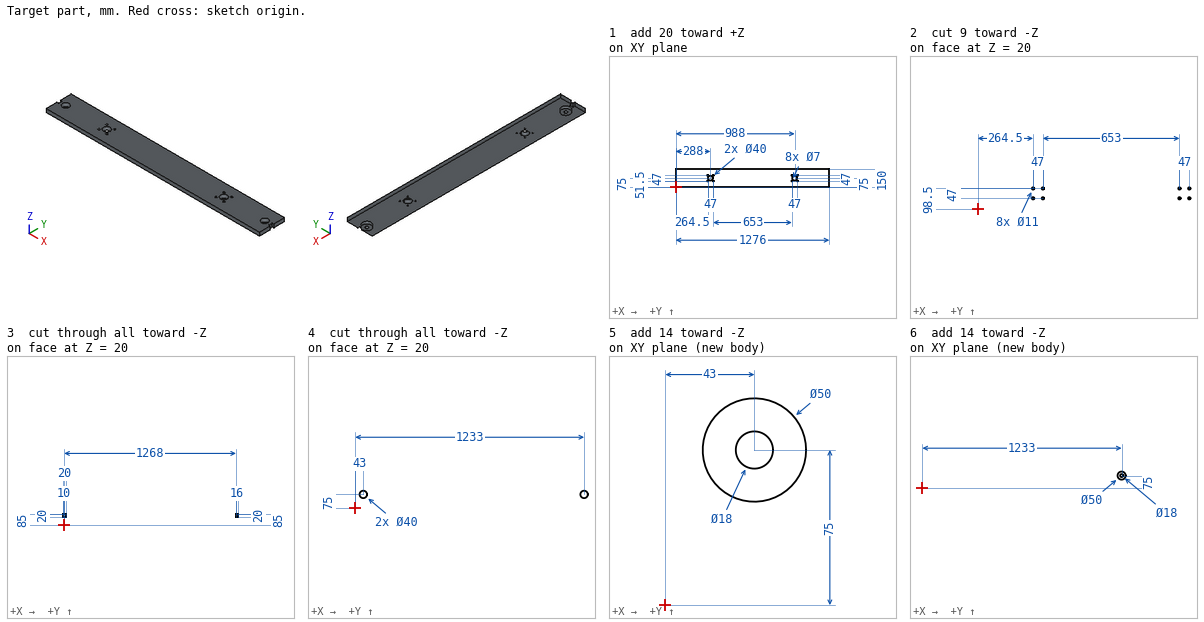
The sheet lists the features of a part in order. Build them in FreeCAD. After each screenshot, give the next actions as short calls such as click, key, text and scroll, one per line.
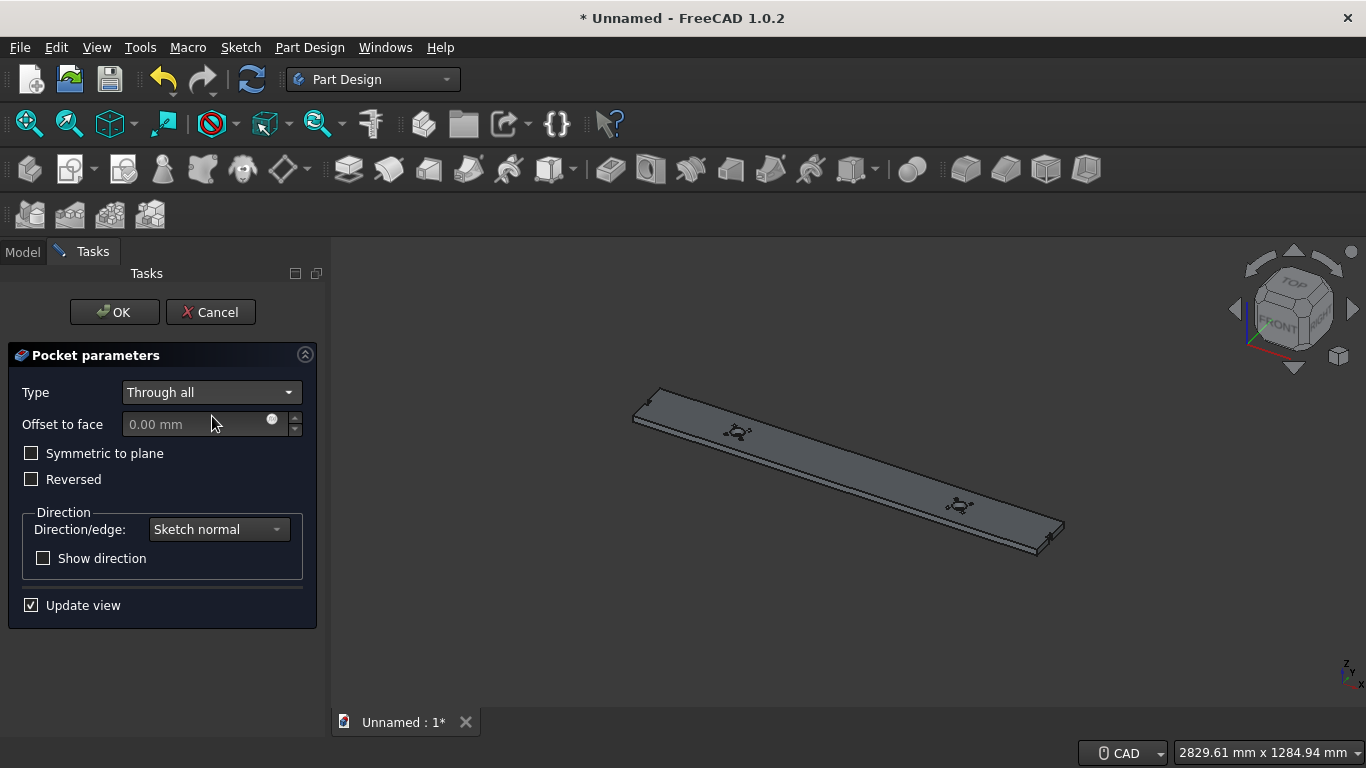
click(115, 312)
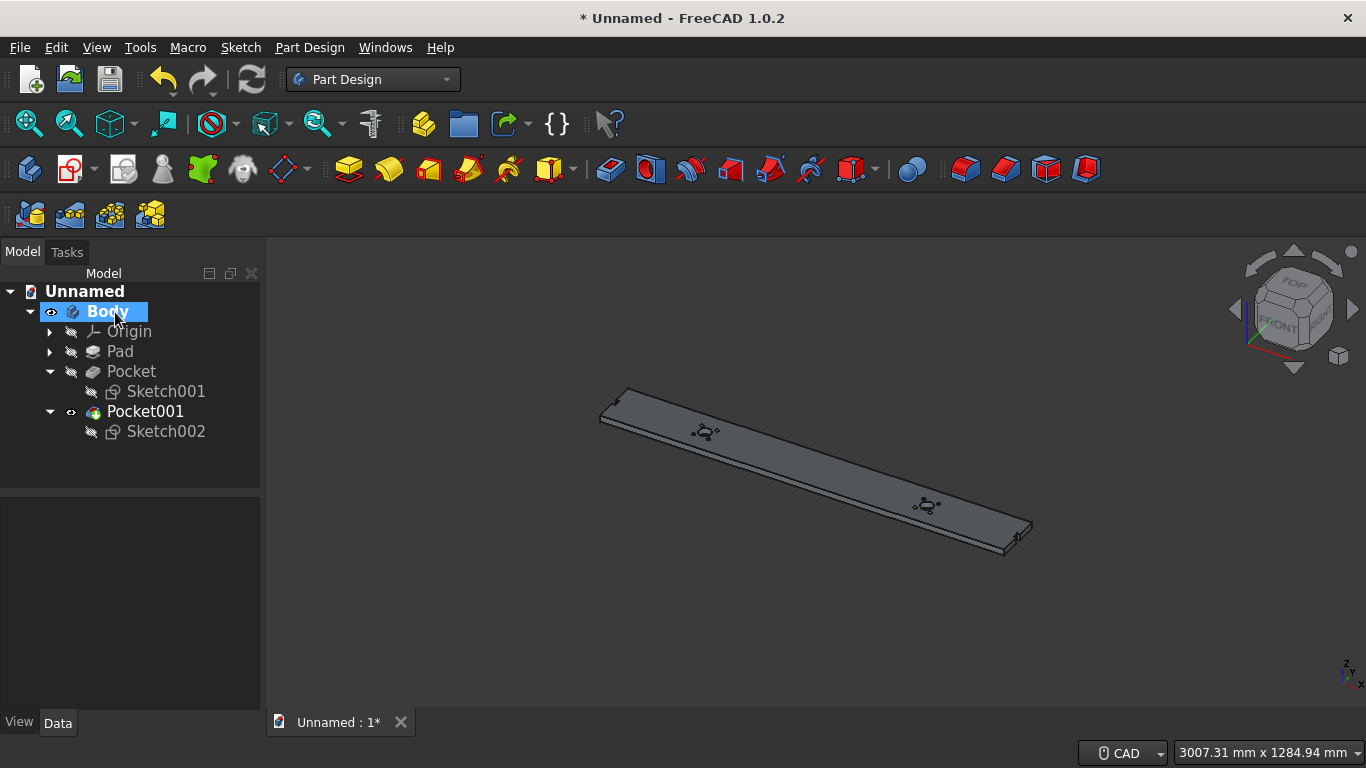
click(30, 124)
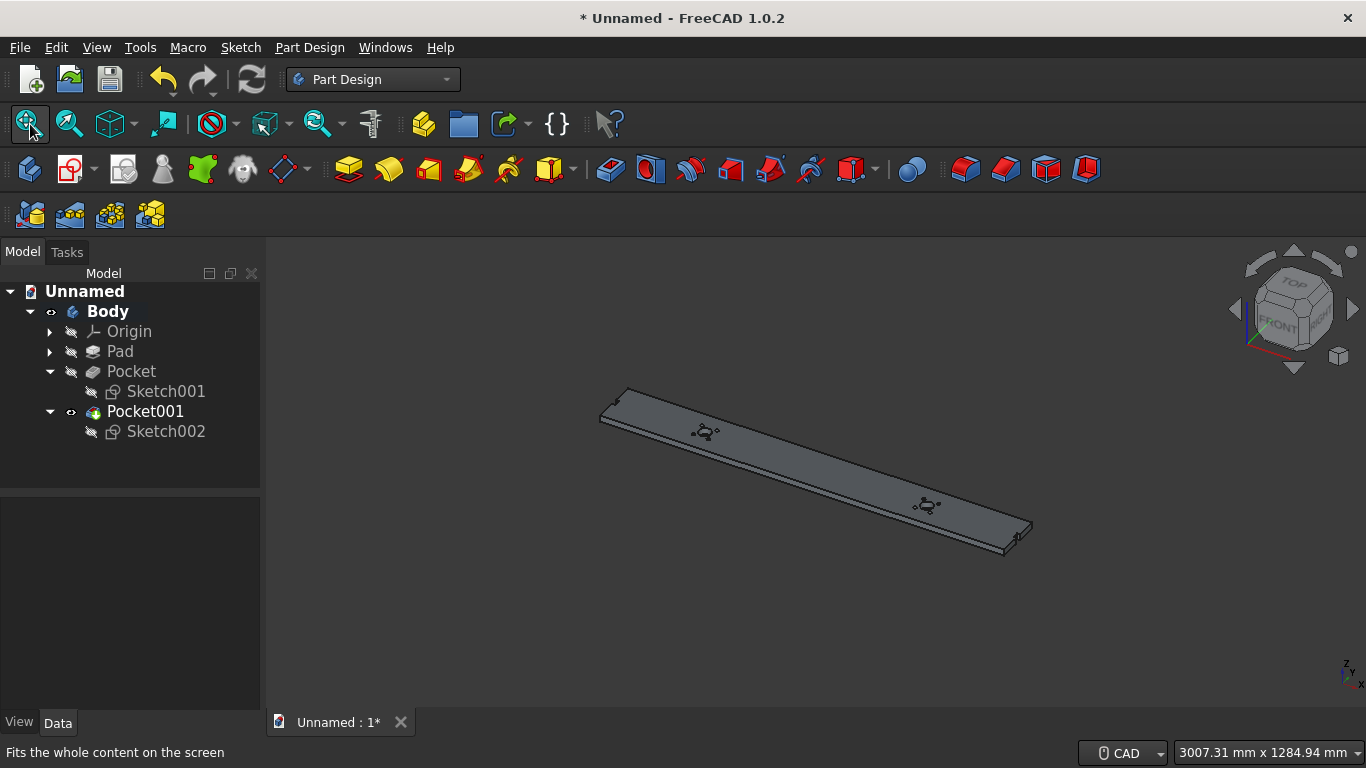
click(989, 525)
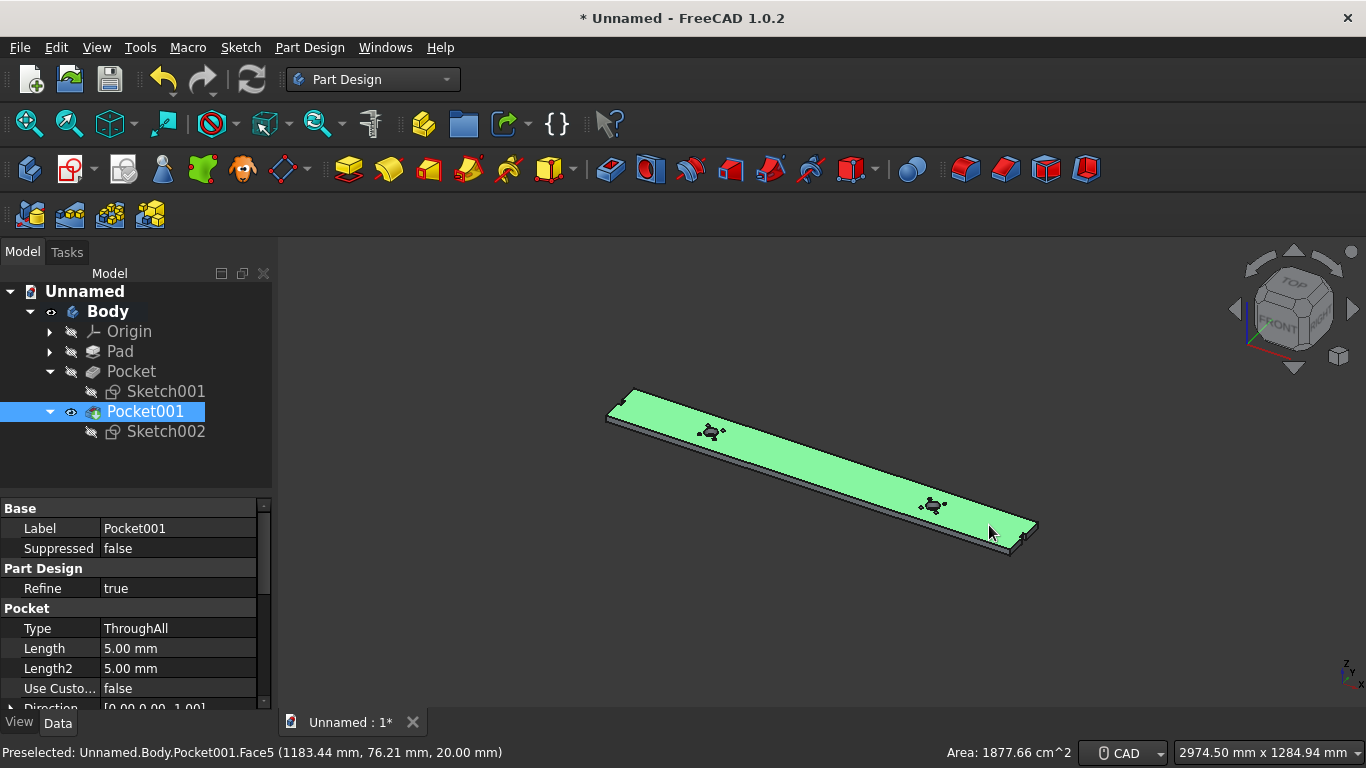
click(70, 170)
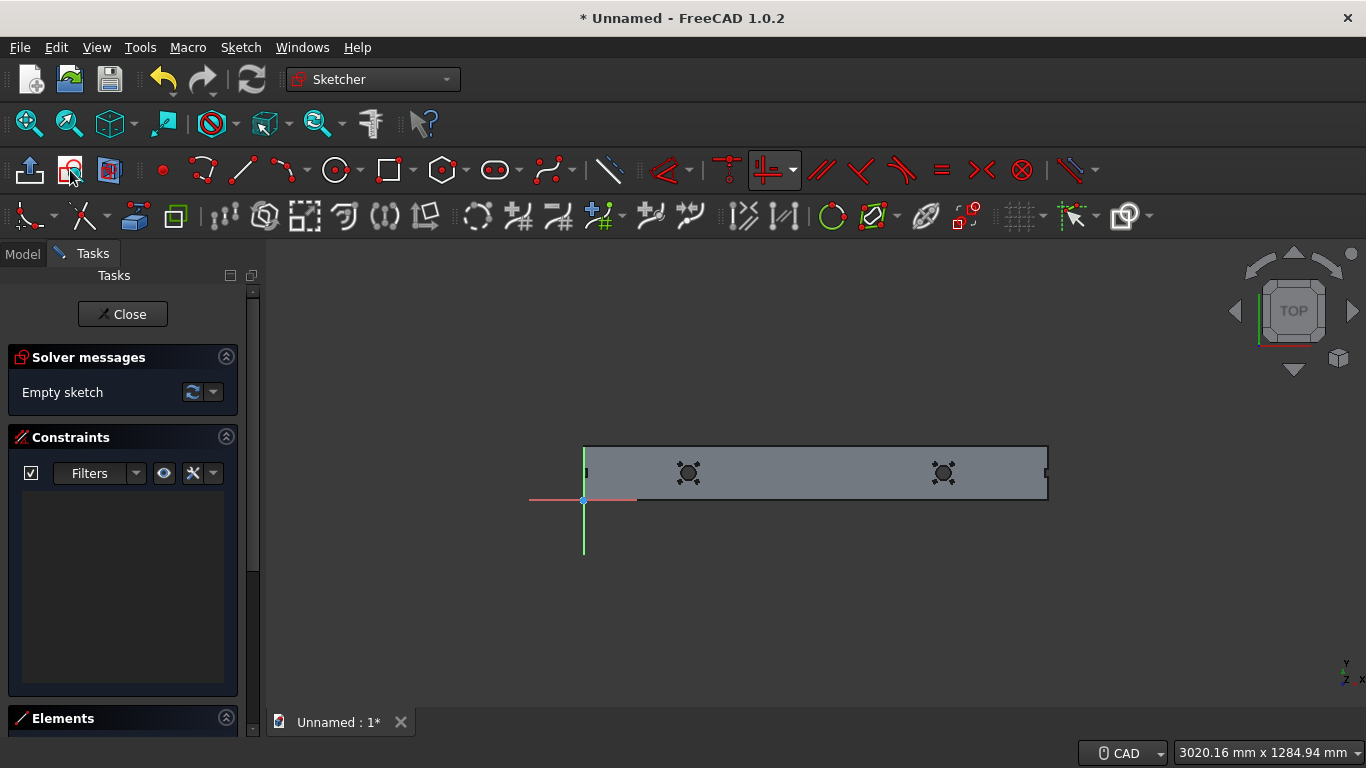
scroll(943, 503, up, 2)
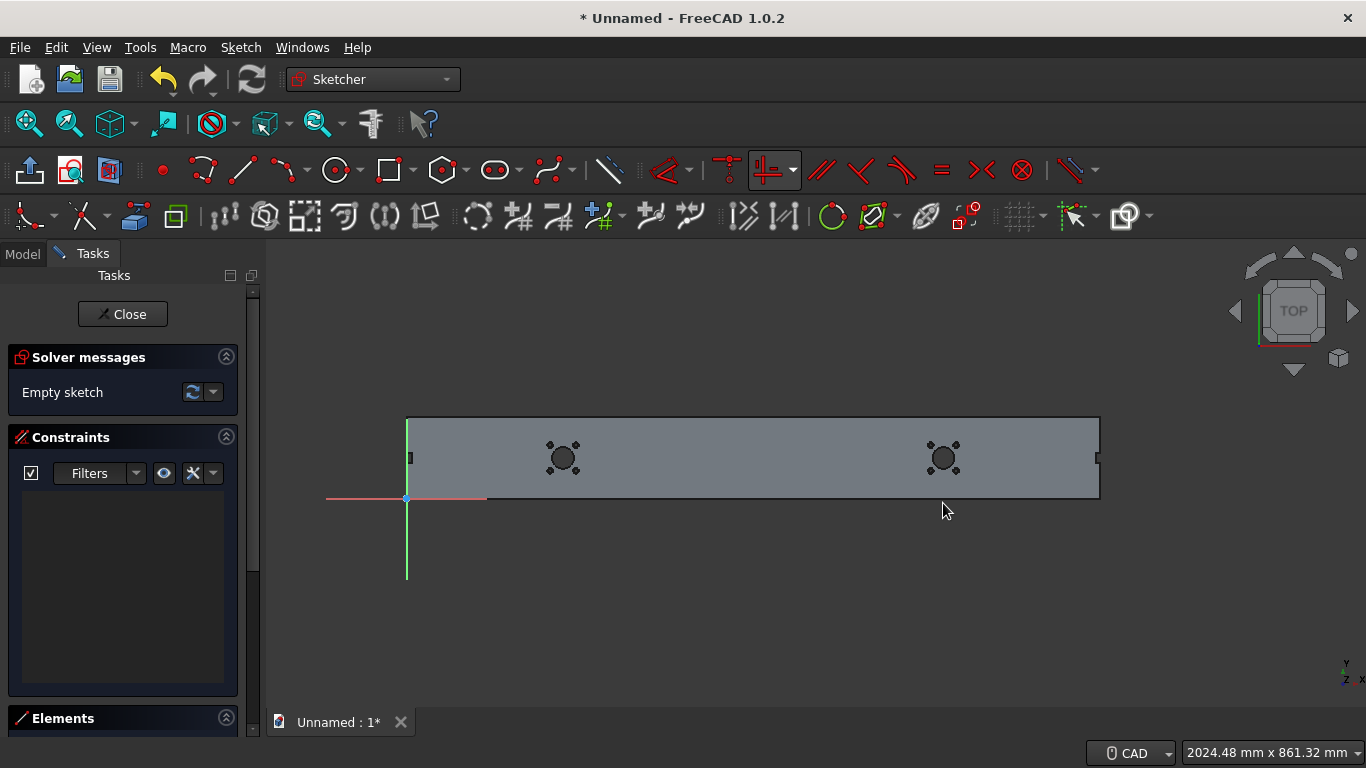
click(336, 170)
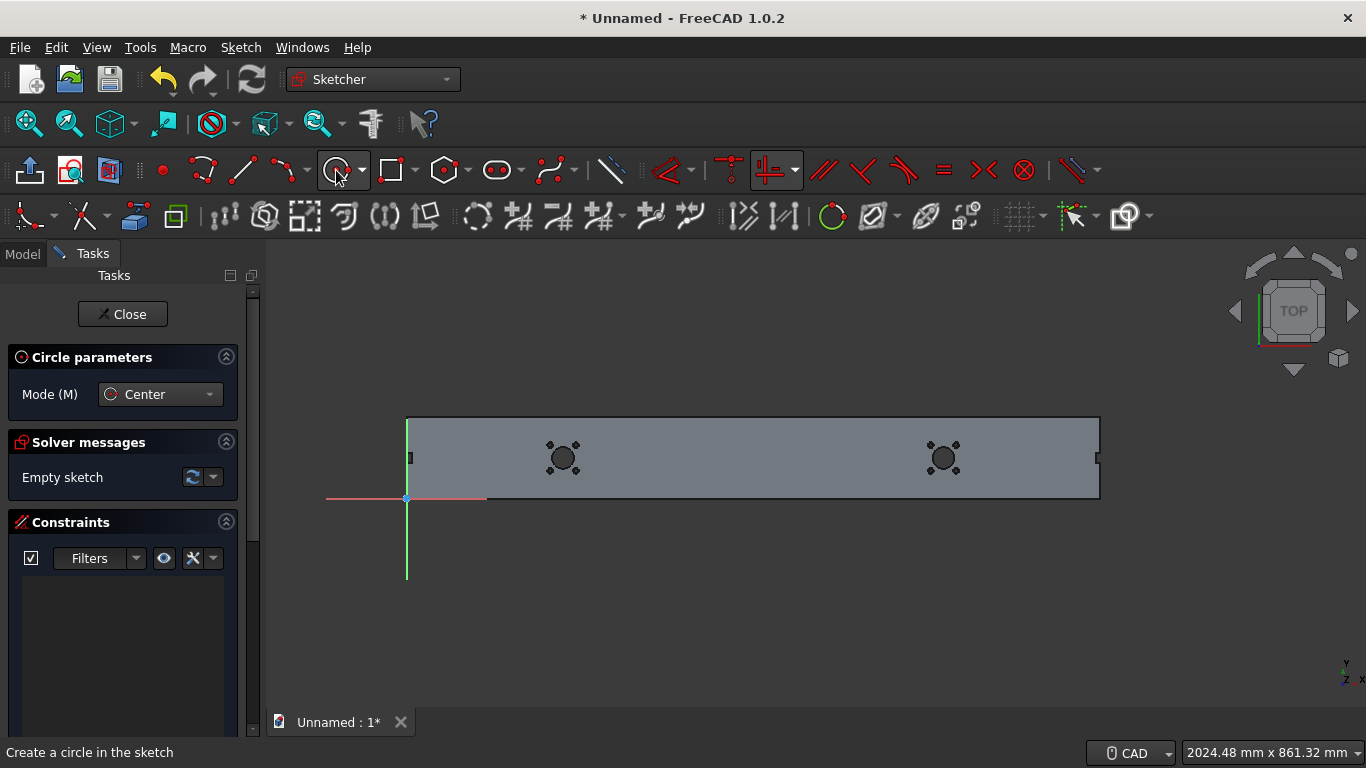
scroll(430, 458, up, 4)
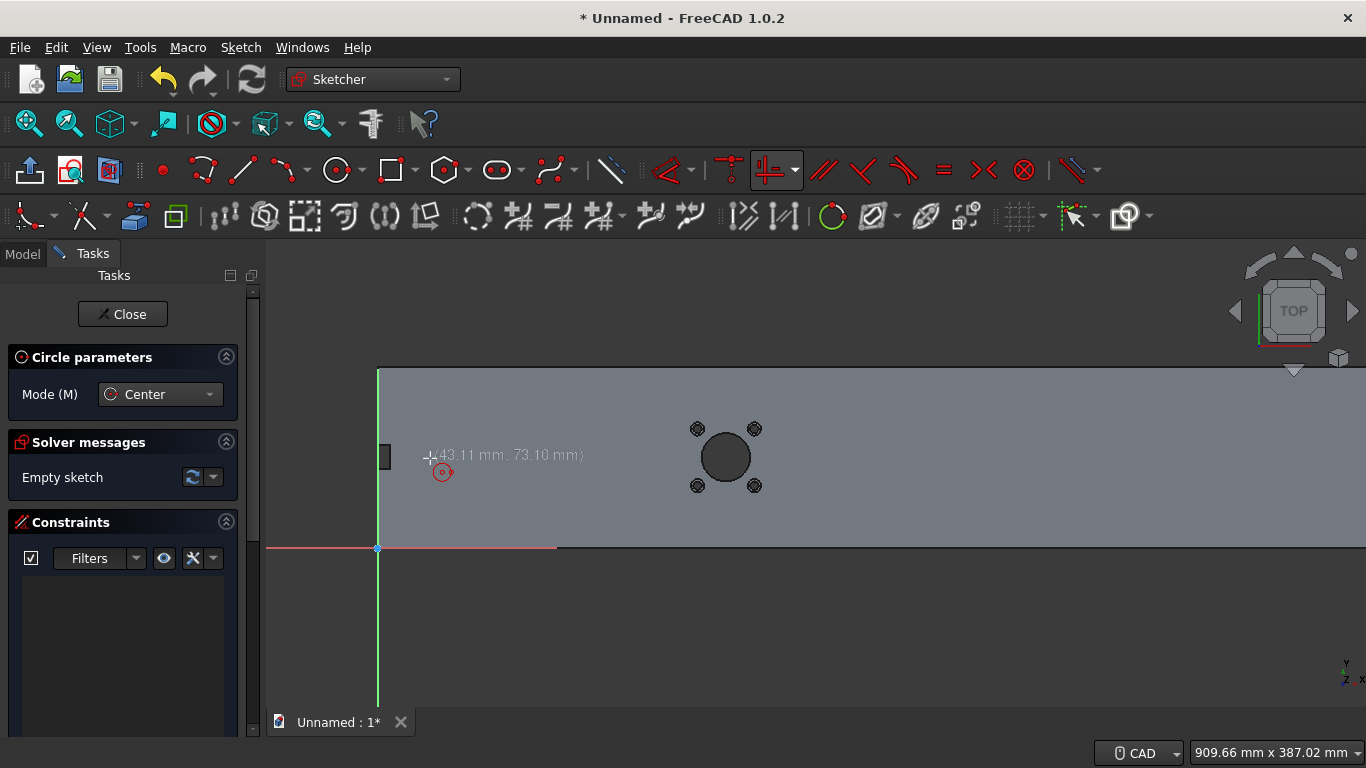
click(430, 457)
move(447, 440)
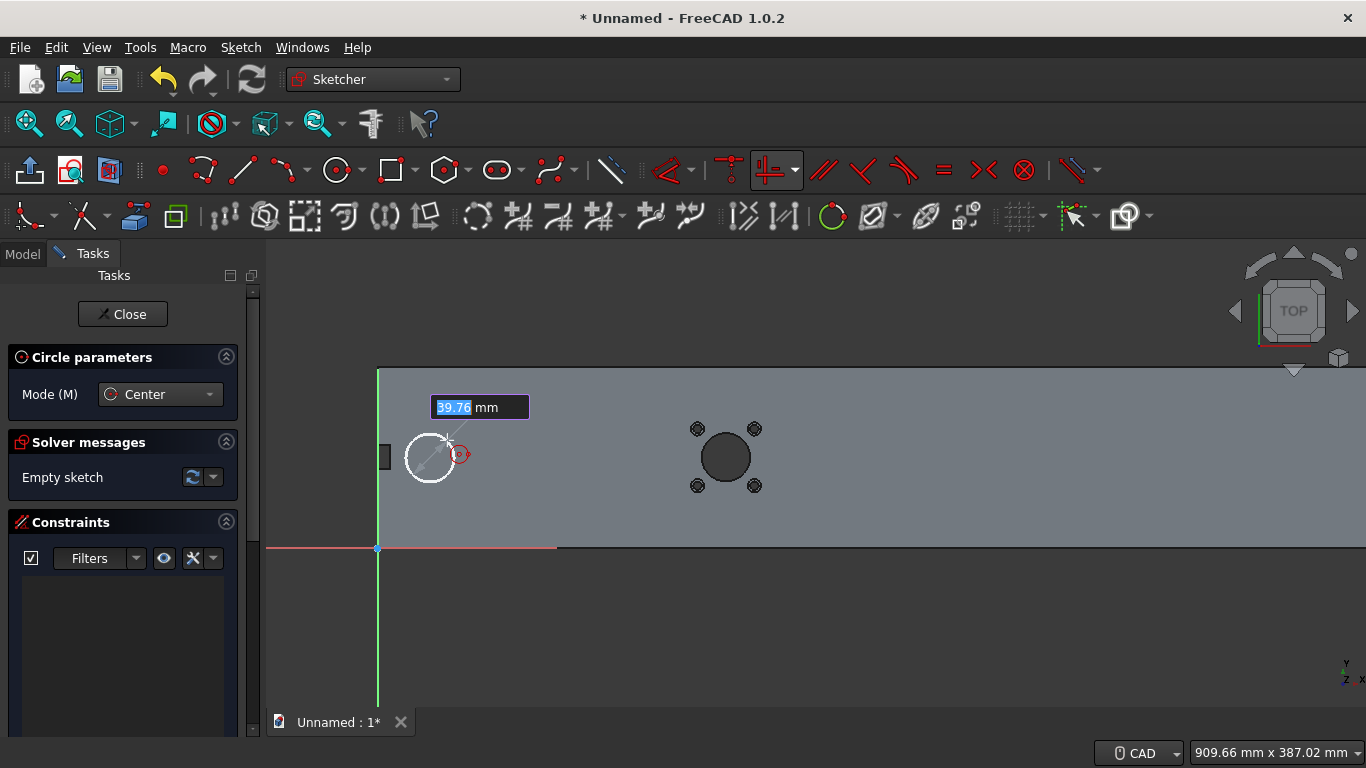
text(40)
key(Return)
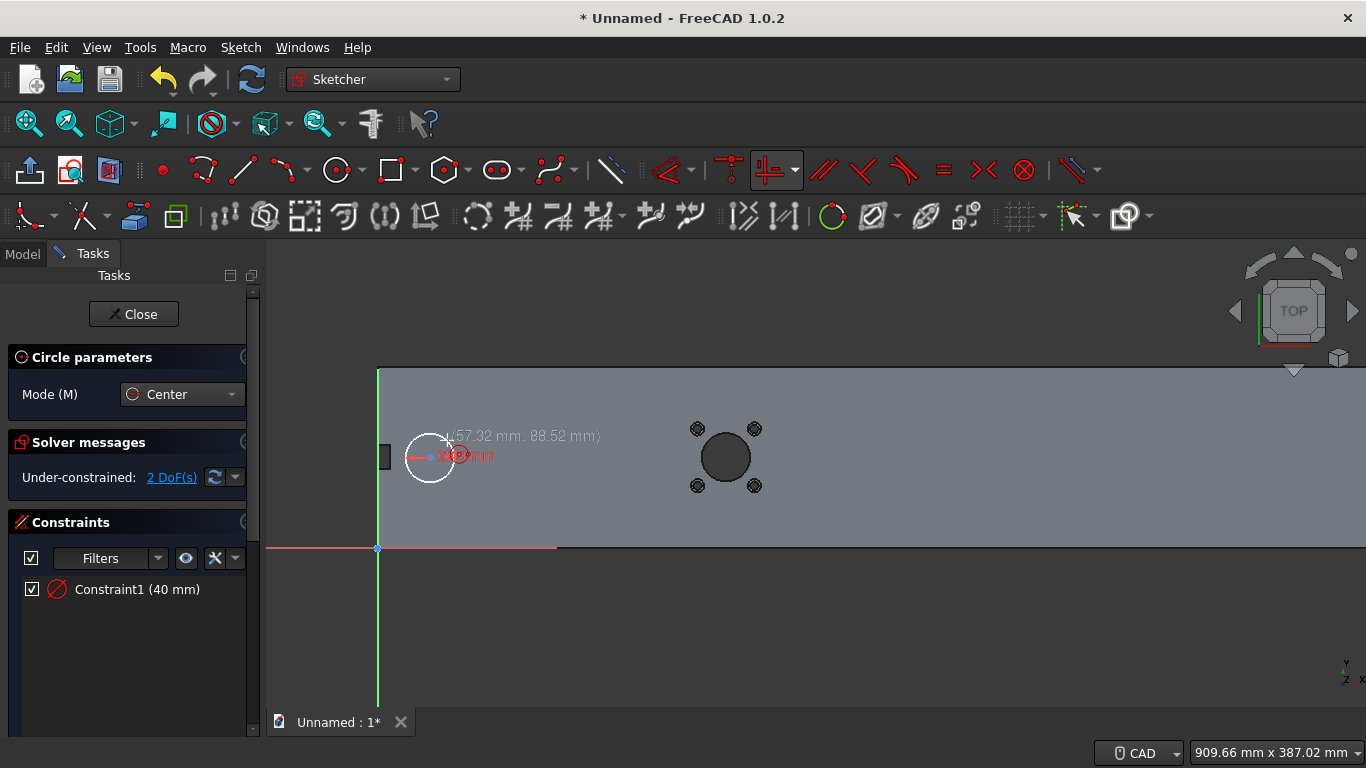
scroll(431, 459, down, 4)